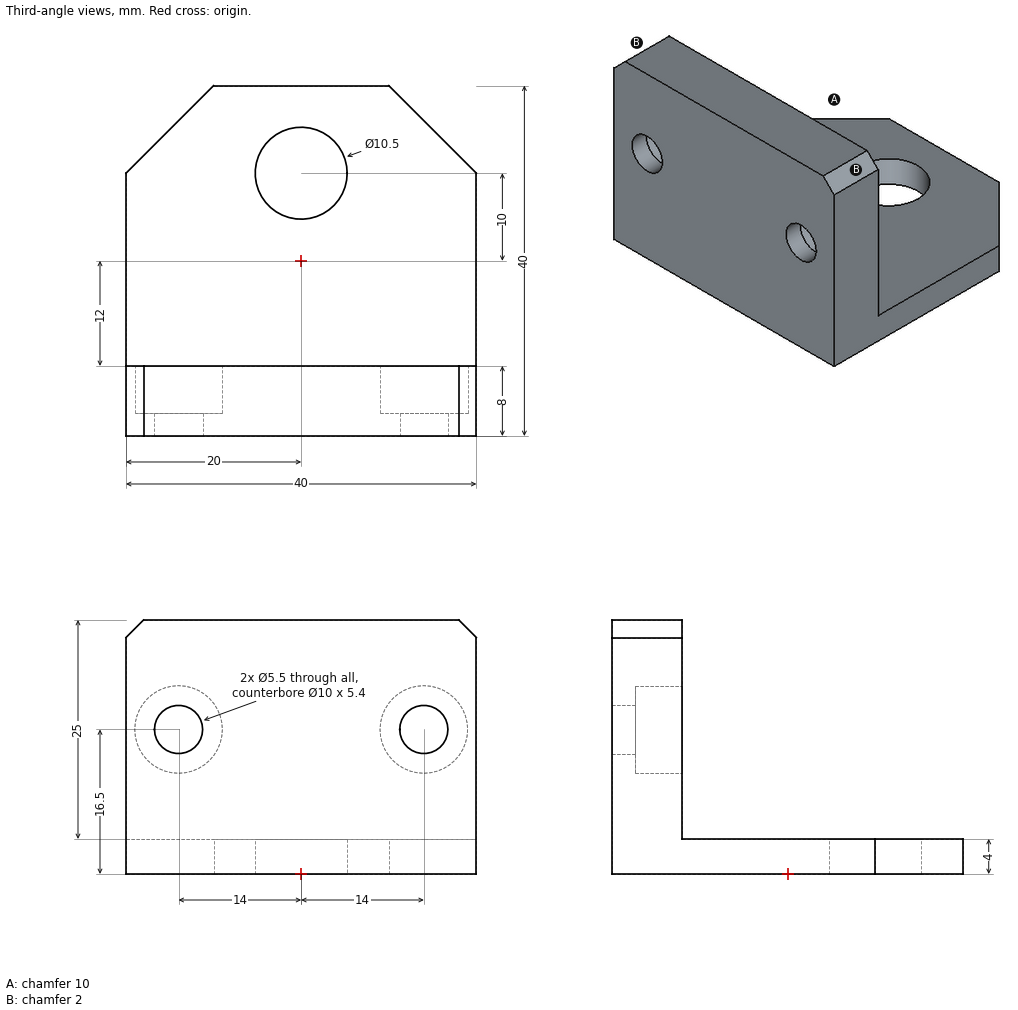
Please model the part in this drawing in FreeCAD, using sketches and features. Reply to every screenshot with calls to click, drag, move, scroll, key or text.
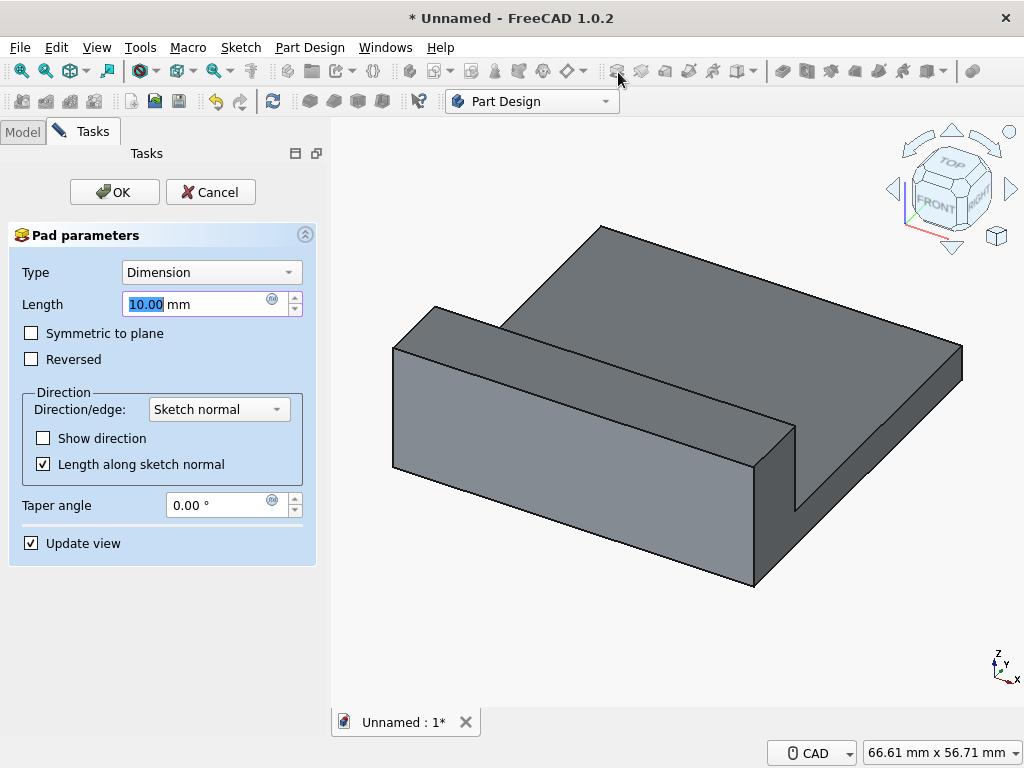
text(25)
key(Tab)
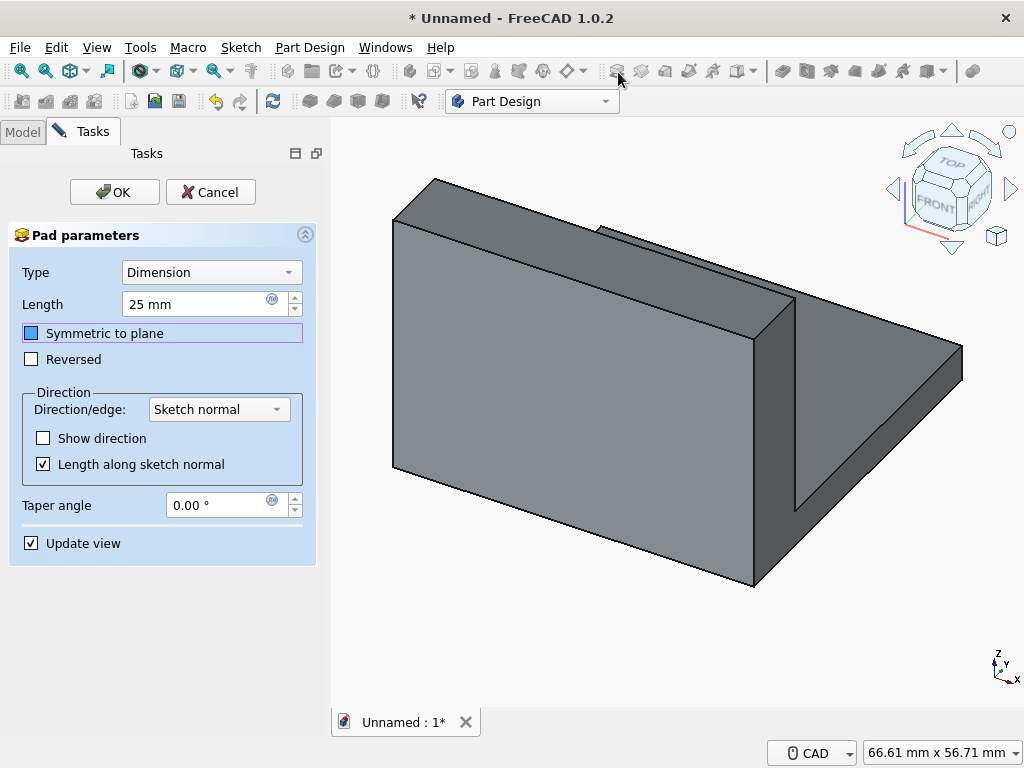
click(115, 192)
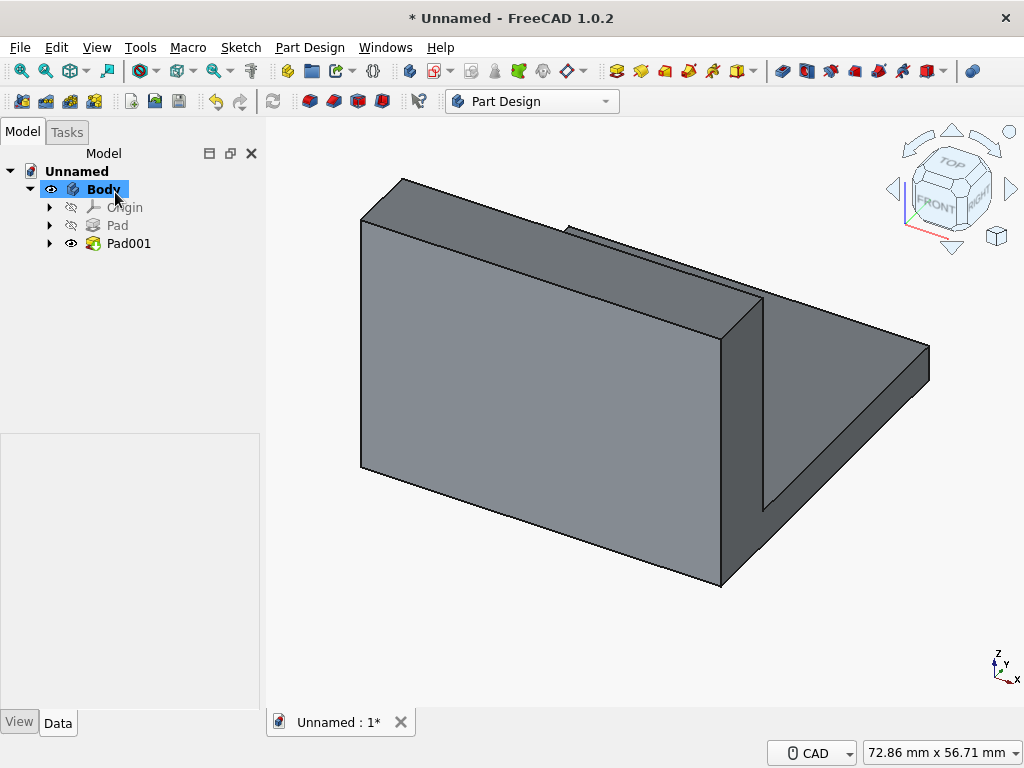
click(22, 72)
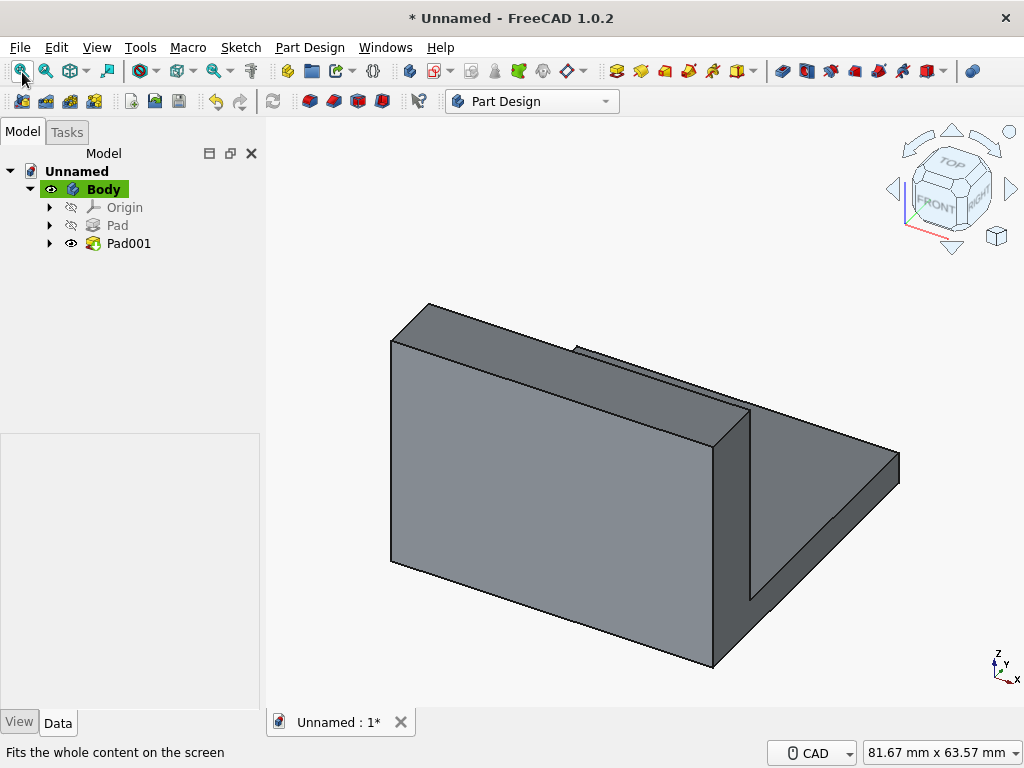
key(0)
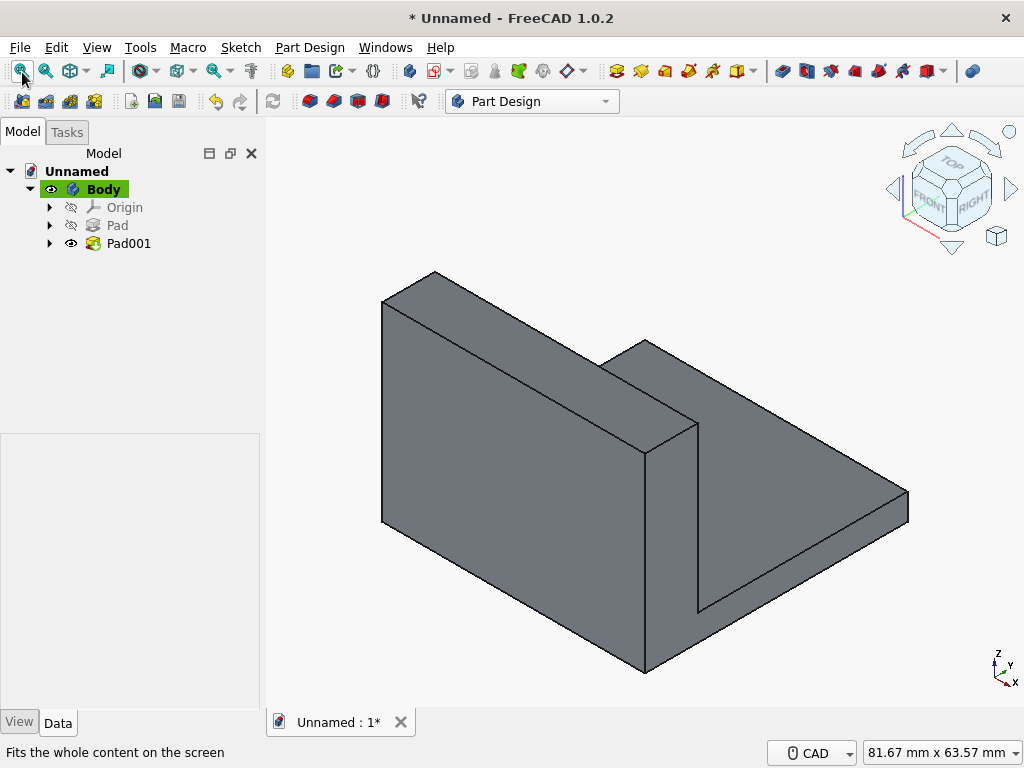
click(709, 497)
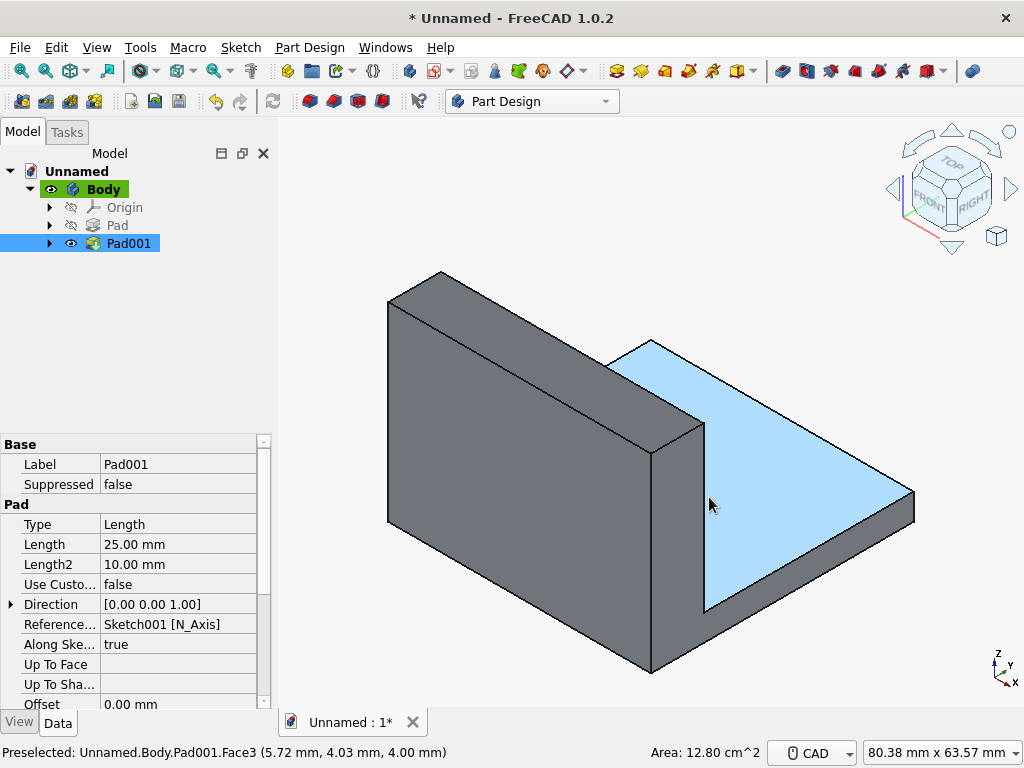
click(434, 72)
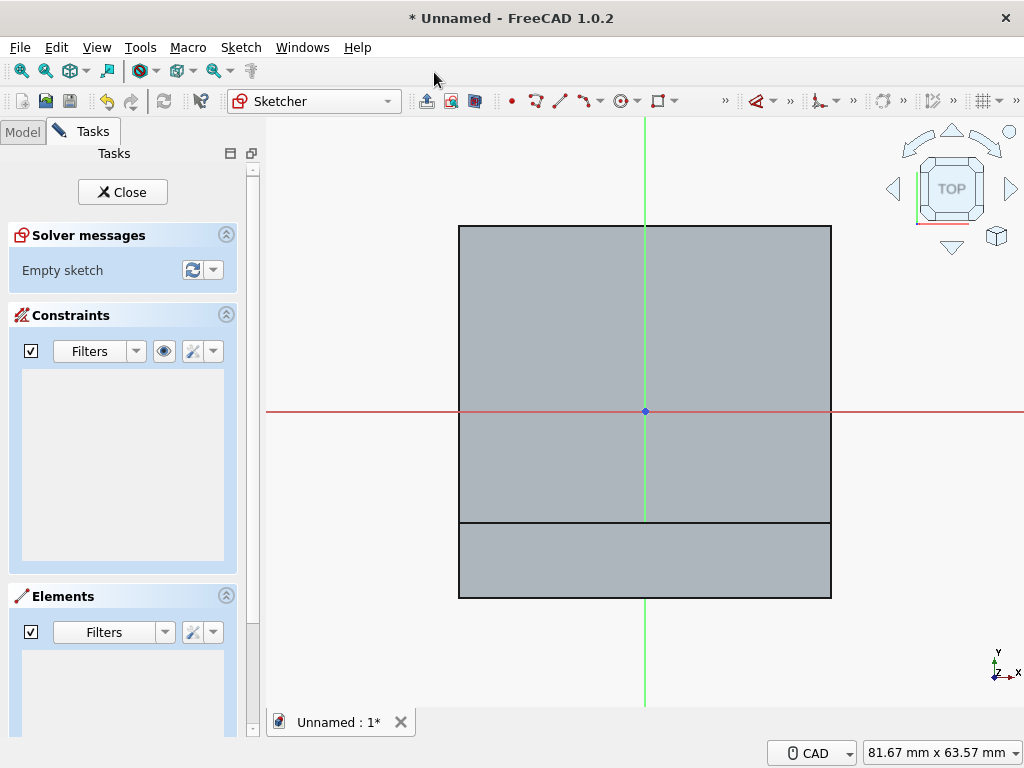
click(476, 102)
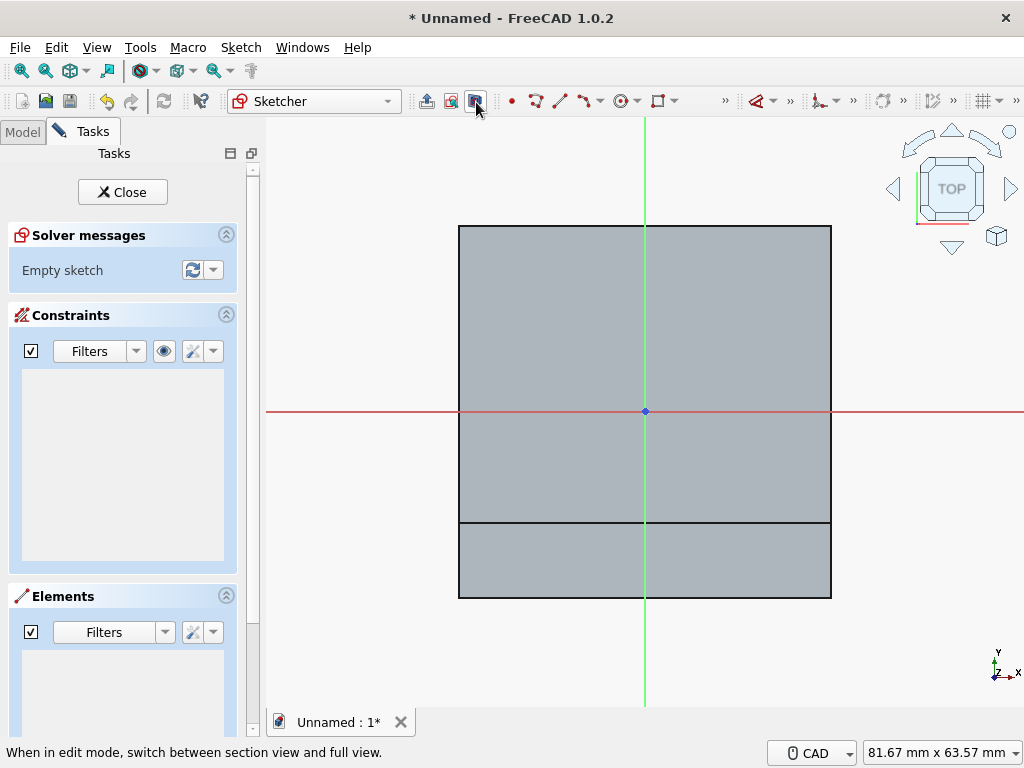
scroll(685, 300, up, 5)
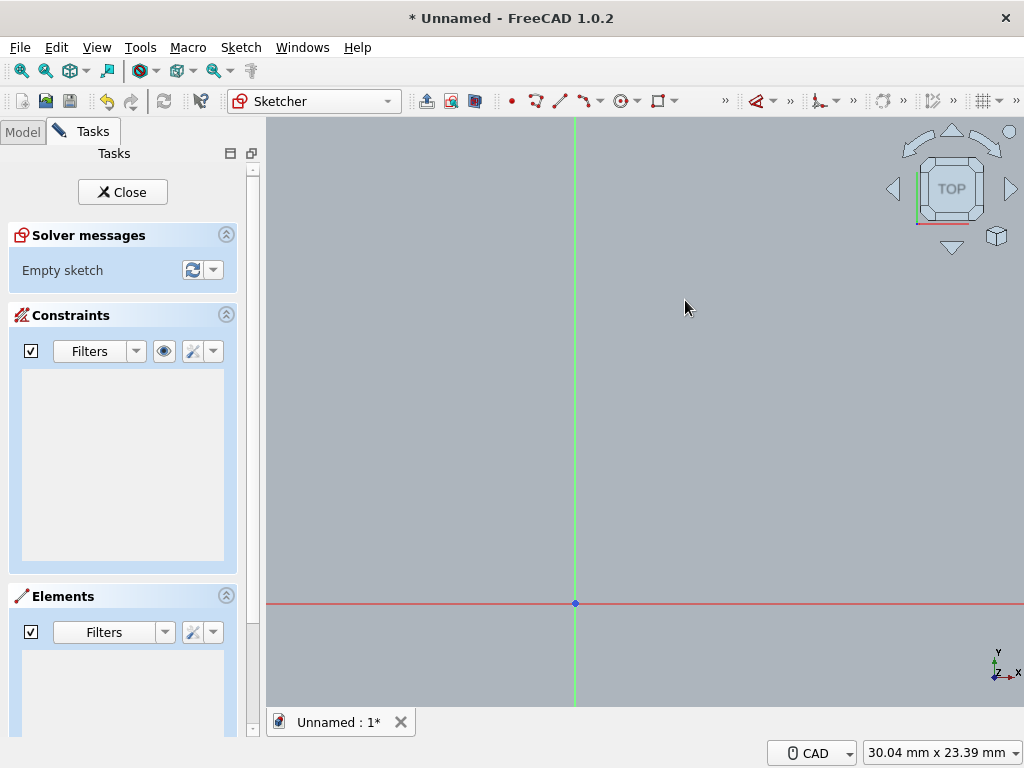
click(622, 102)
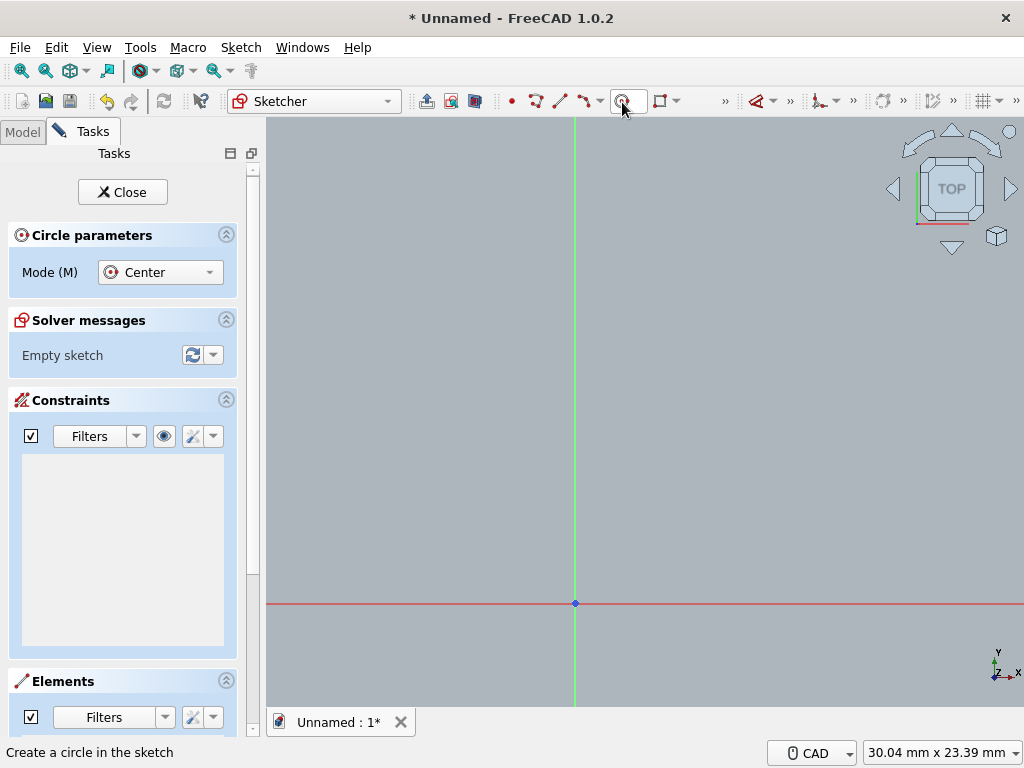
click(575, 352)
move(669, 258)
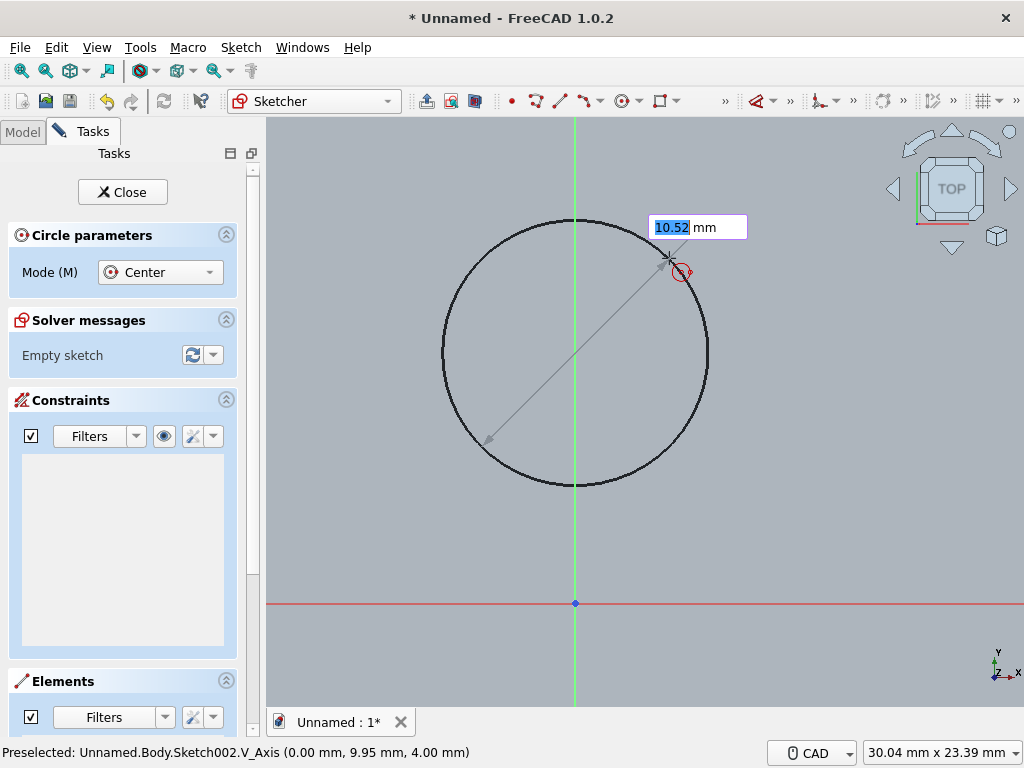
text(10.5)
key(Return)
key(Escape)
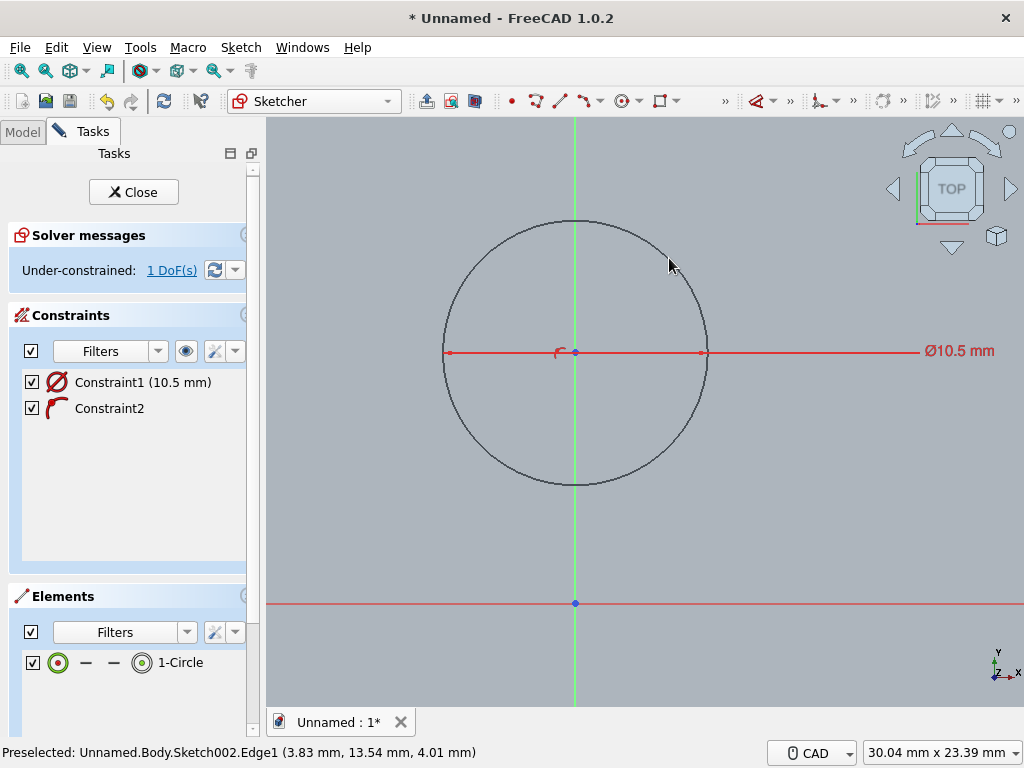
key(d)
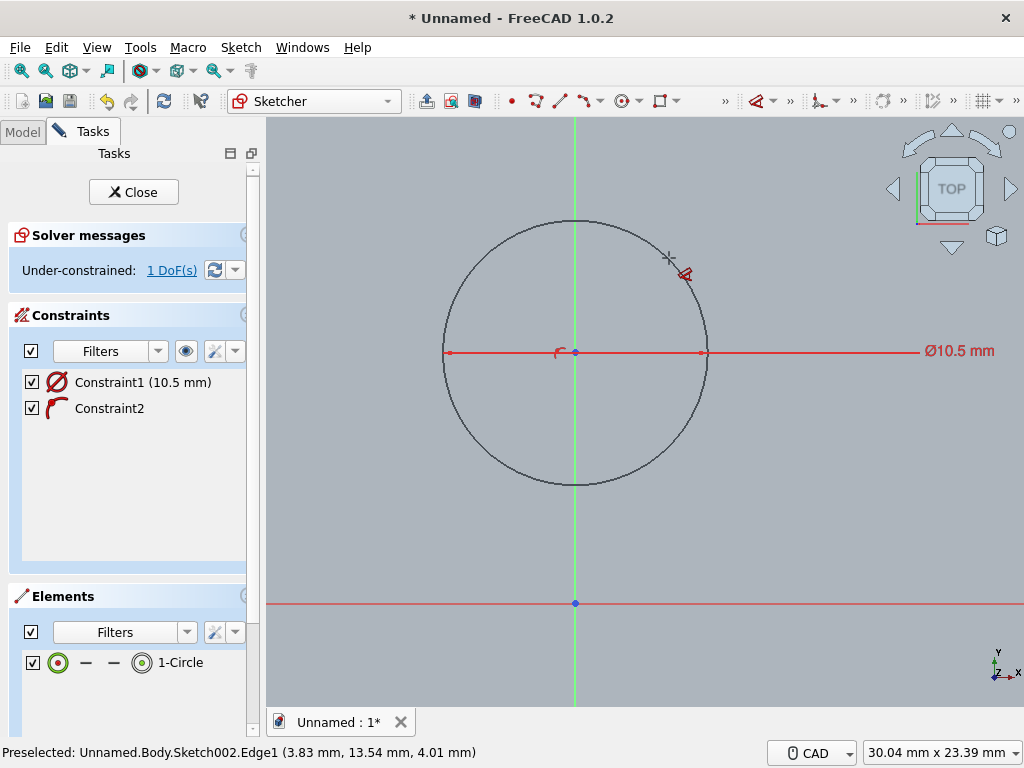
click(575, 353)
click(609, 421)